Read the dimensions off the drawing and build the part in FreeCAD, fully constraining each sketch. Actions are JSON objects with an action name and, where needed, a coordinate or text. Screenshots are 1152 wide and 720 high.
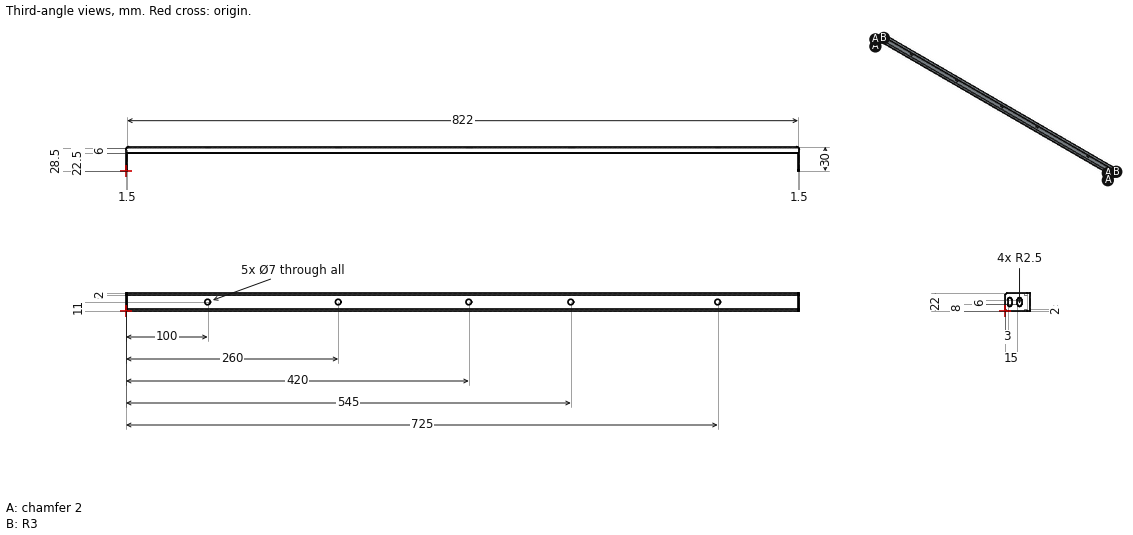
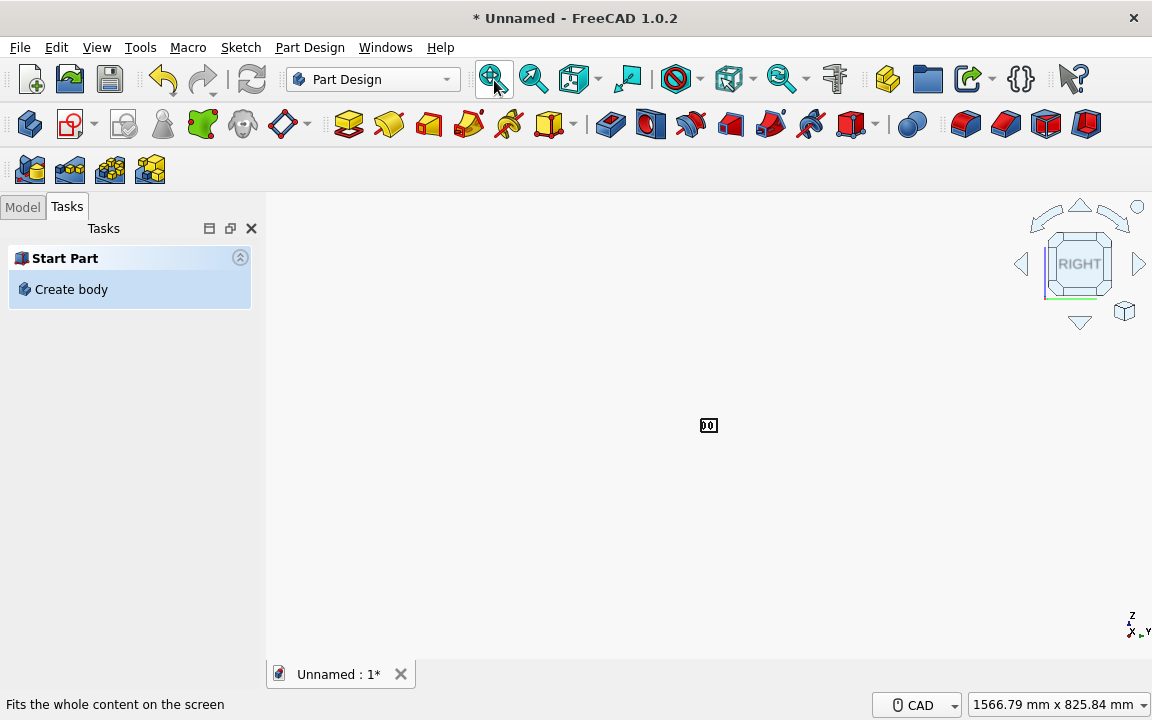
{"action": "left_click", "coordinate": [494, 80]}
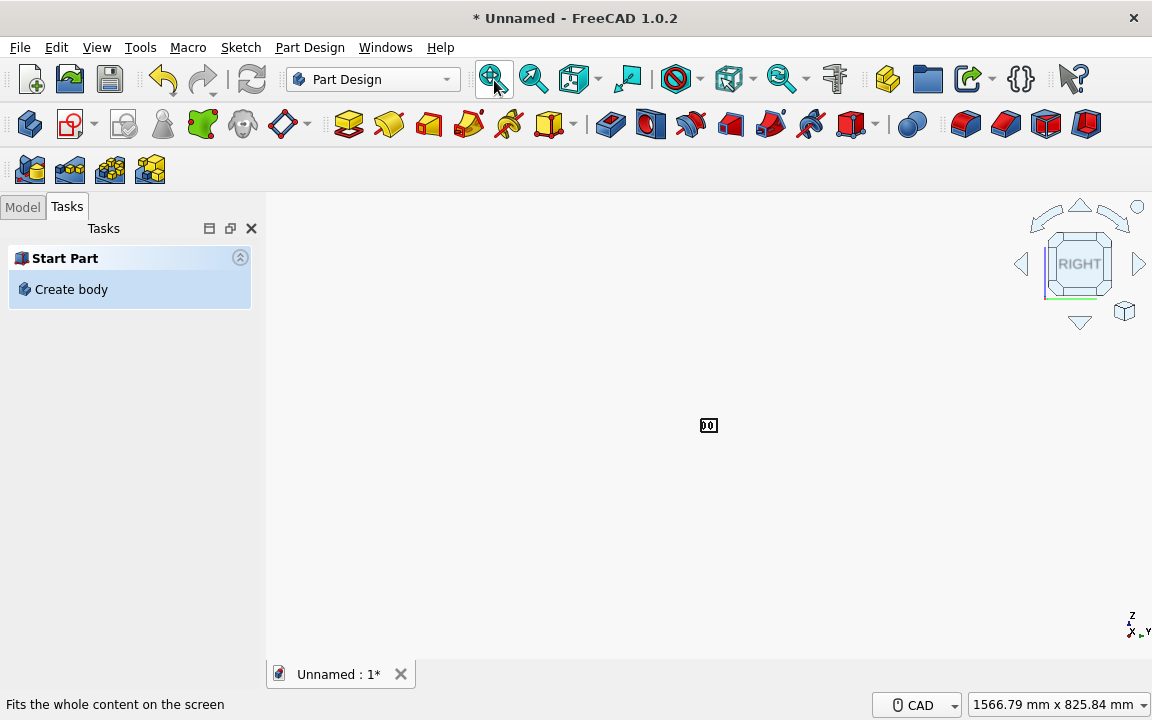
{"action": "scroll", "coordinate": [717, 424], "scroll_direction": "up", "scroll_amount": 6}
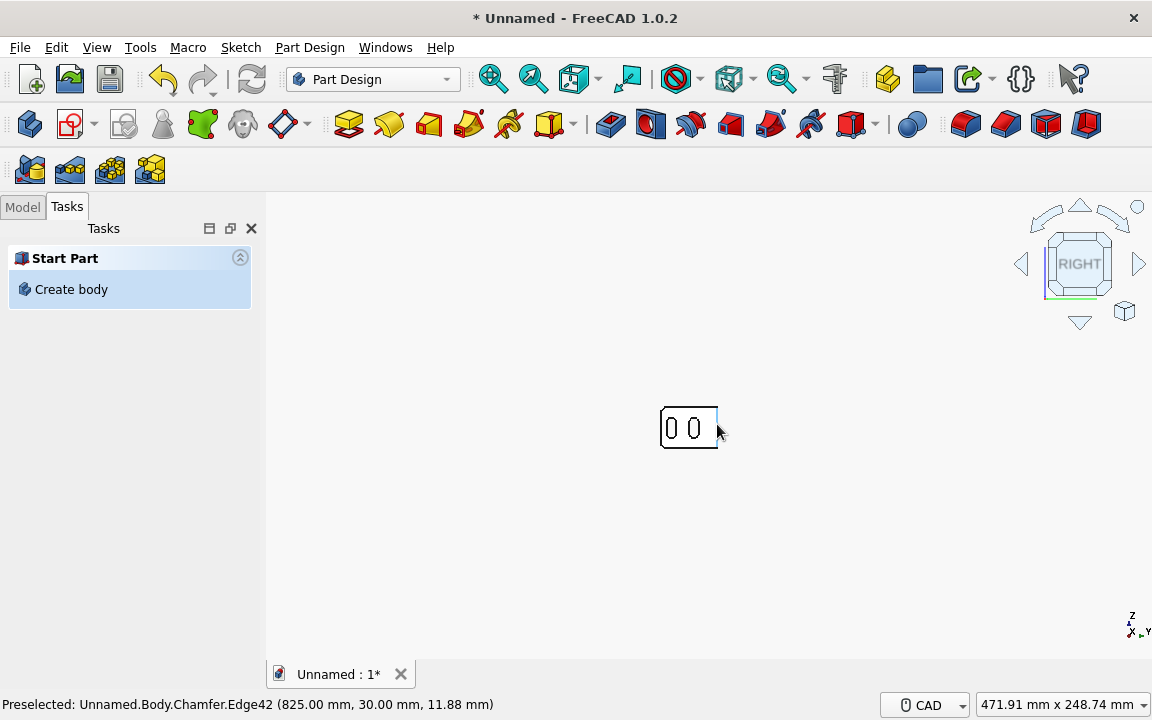
{"action": "left_click", "coordinate": [717, 427]}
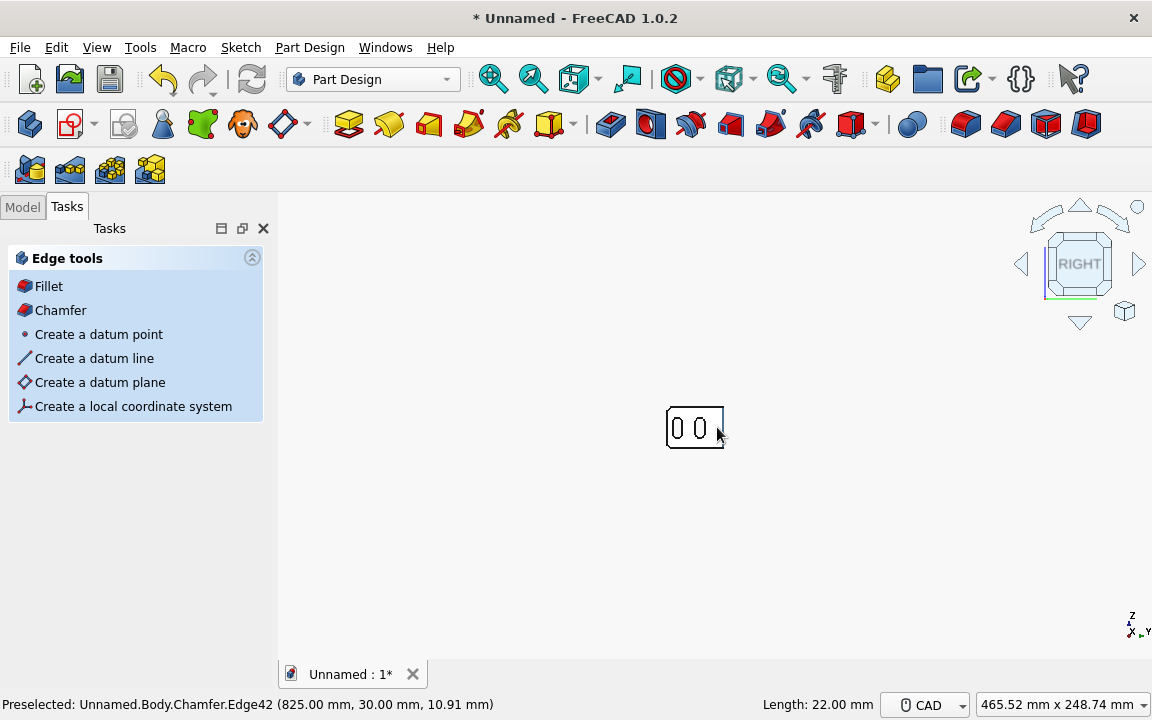
{"action": "left_click", "coordinate": [494, 80]}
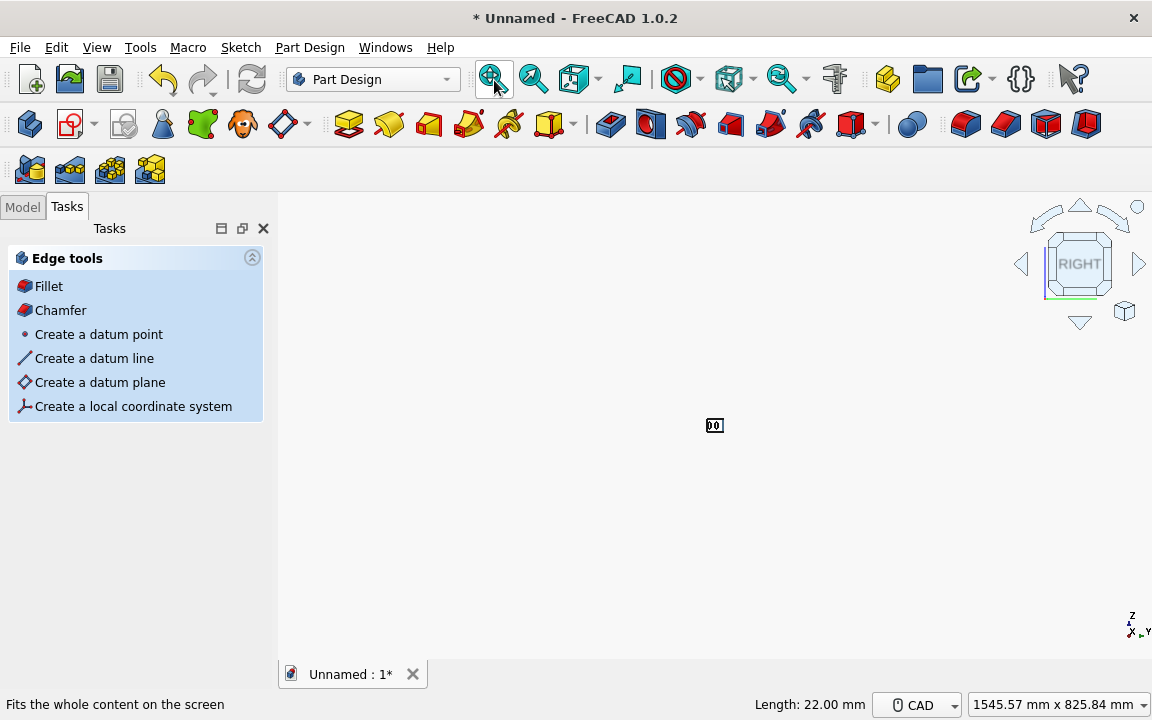
{"action": "key", "text": "5"}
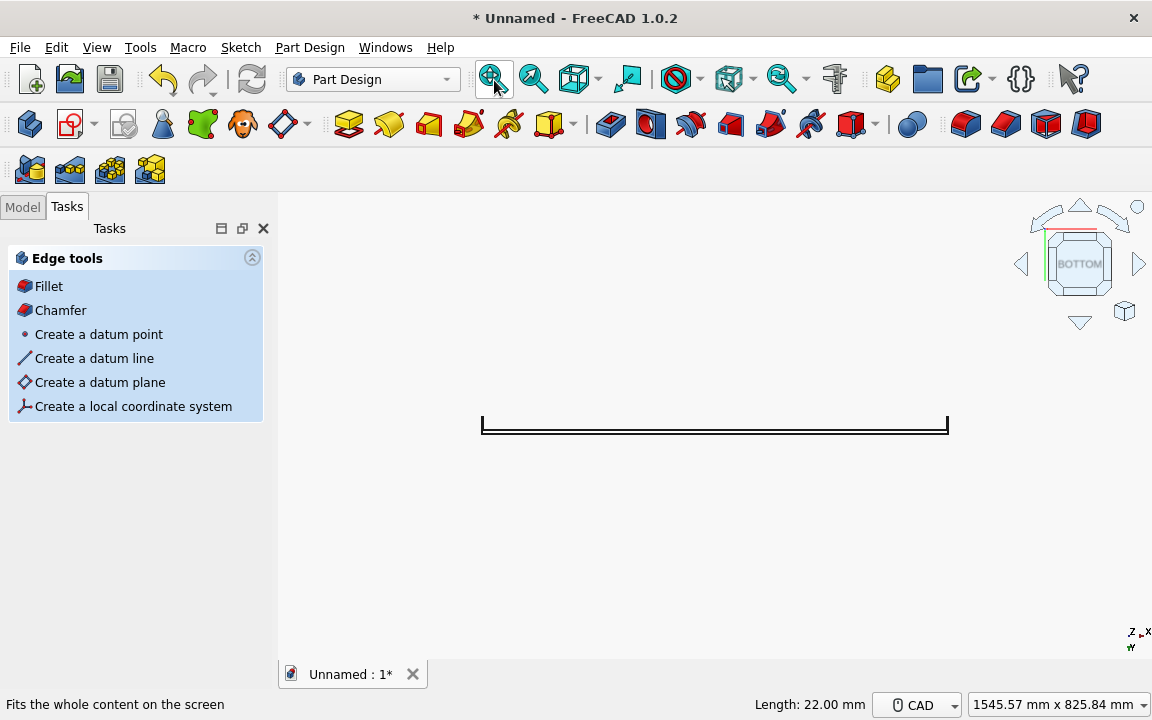
{"action": "scroll", "coordinate": [482, 433], "scroll_direction": "up", "scroll_amount": 6}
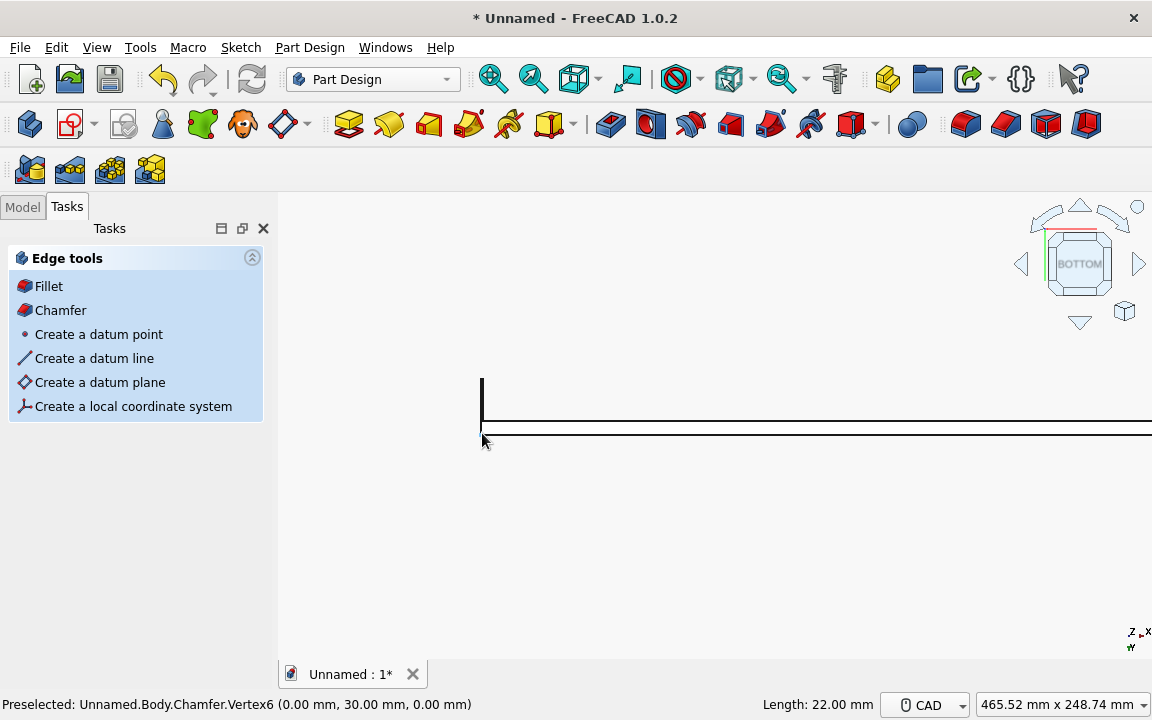
{"action": "left_click", "coordinate": [494, 80]}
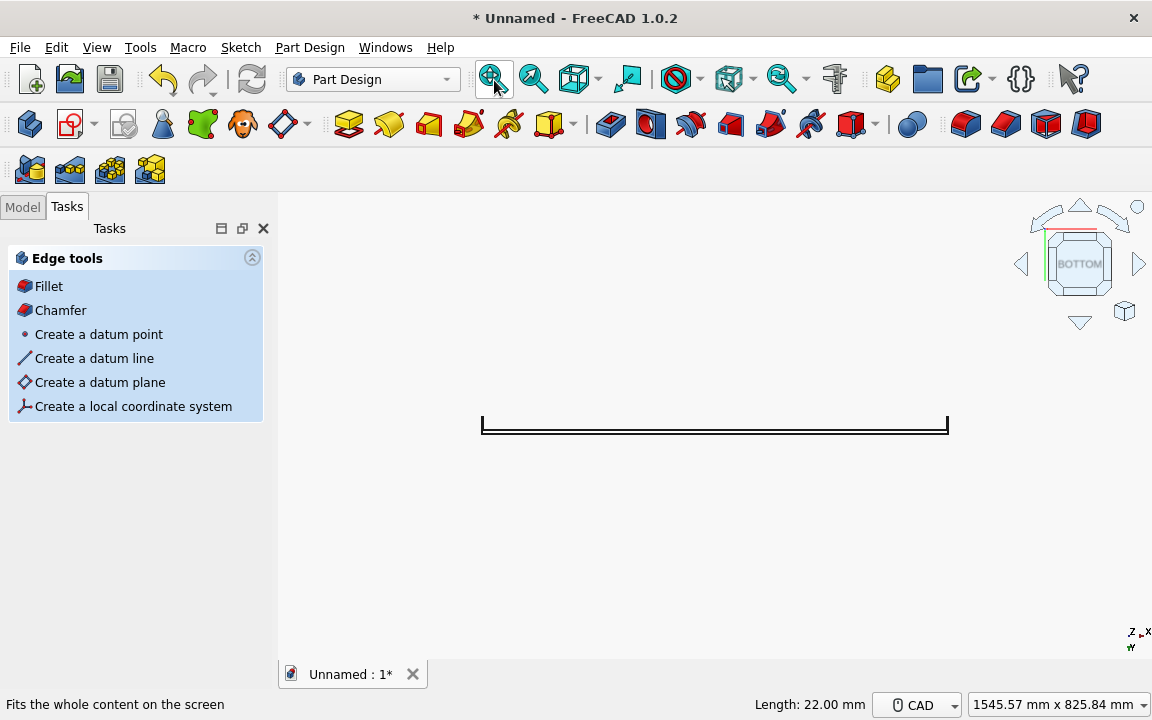
{"action": "key", "text": "4"}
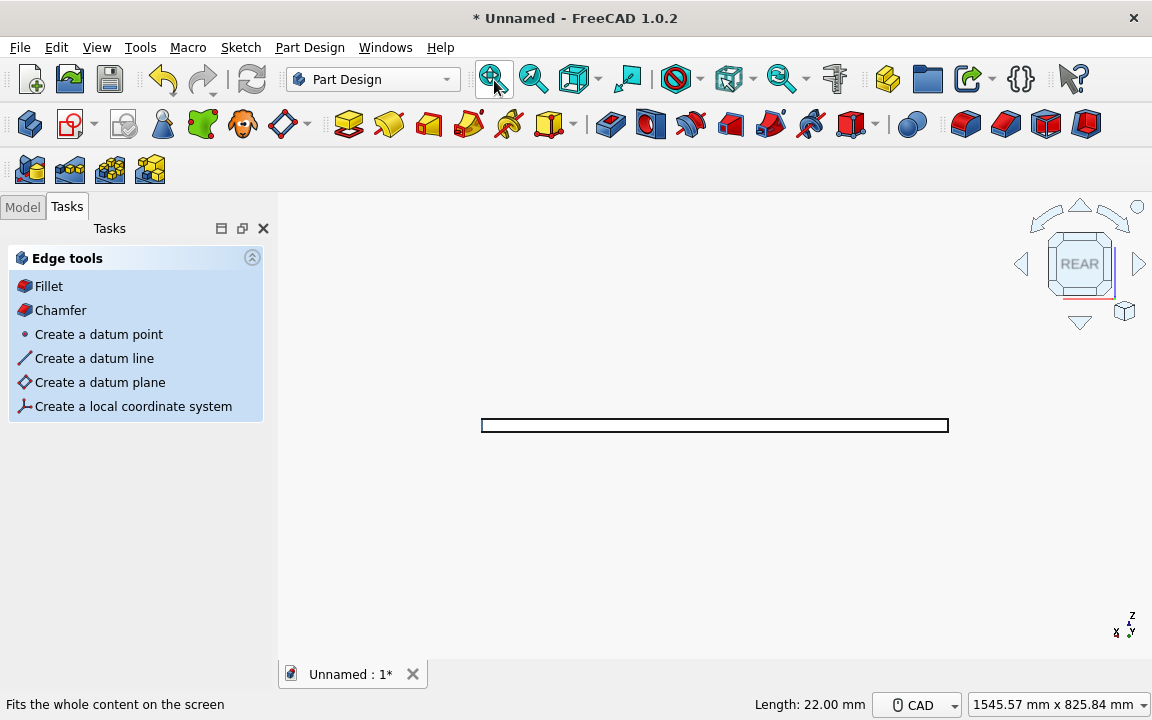
{"action": "scroll", "coordinate": [948, 424], "scroll_direction": "up", "scroll_amount": 6}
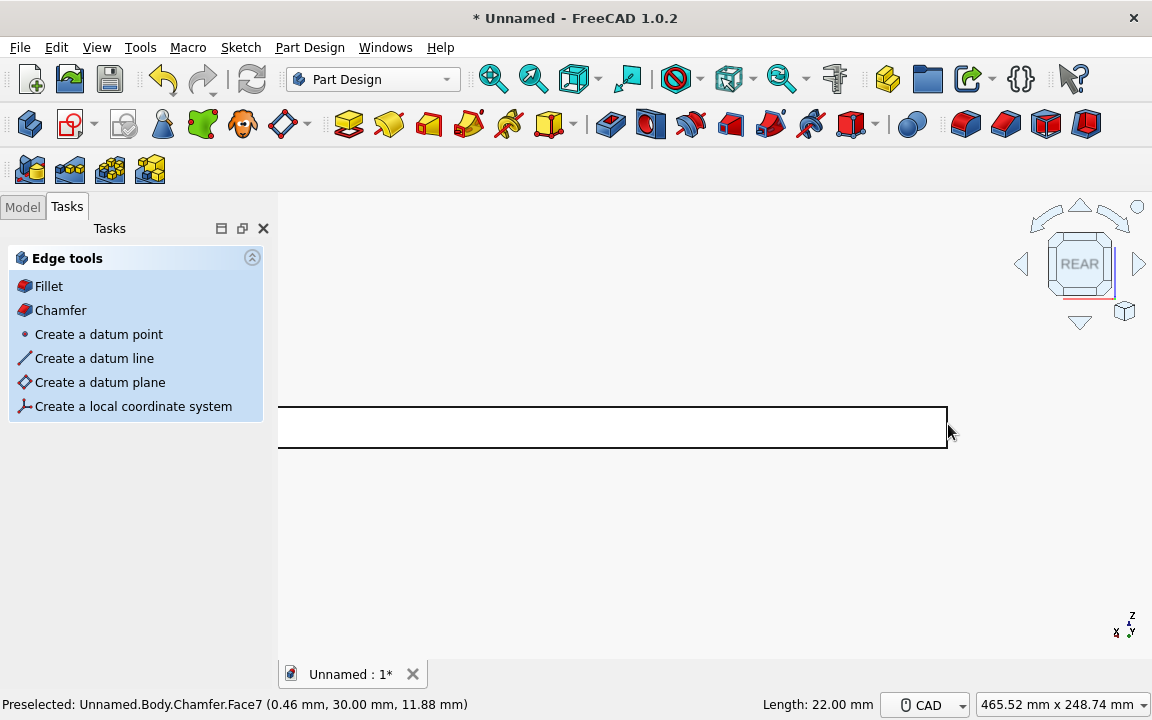
{"action": "left_click", "coordinate": [947, 427], "text": "ctrl"}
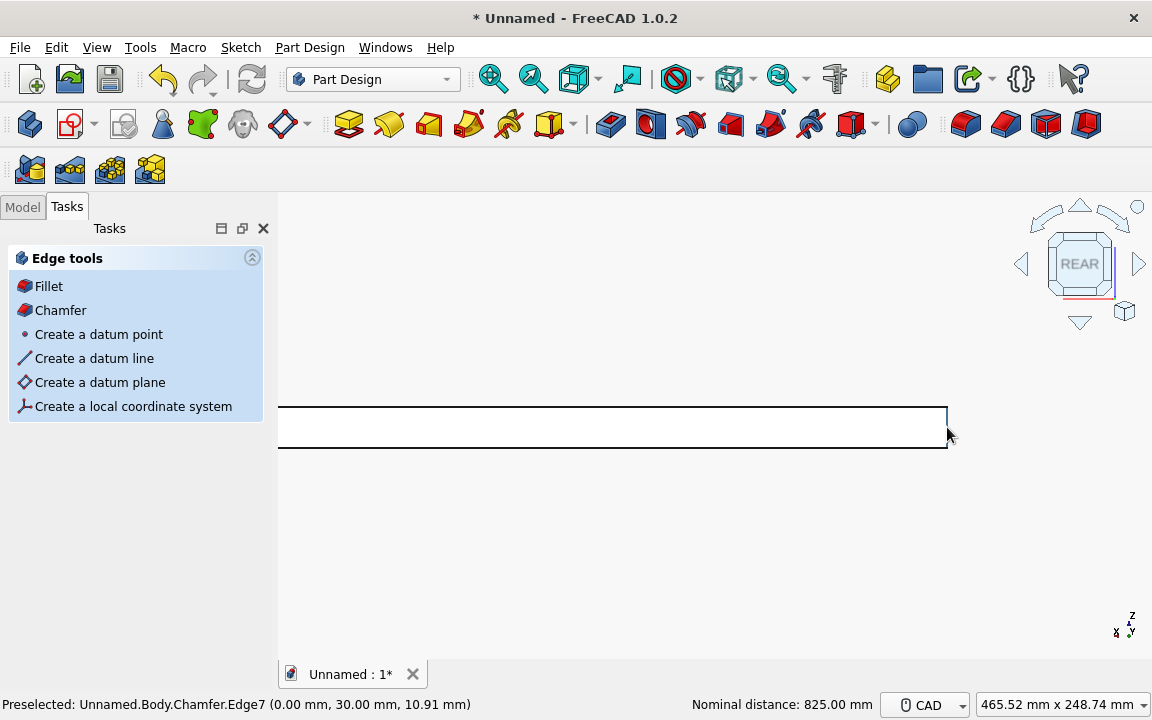
{"action": "left_click", "coordinate": [966, 124]}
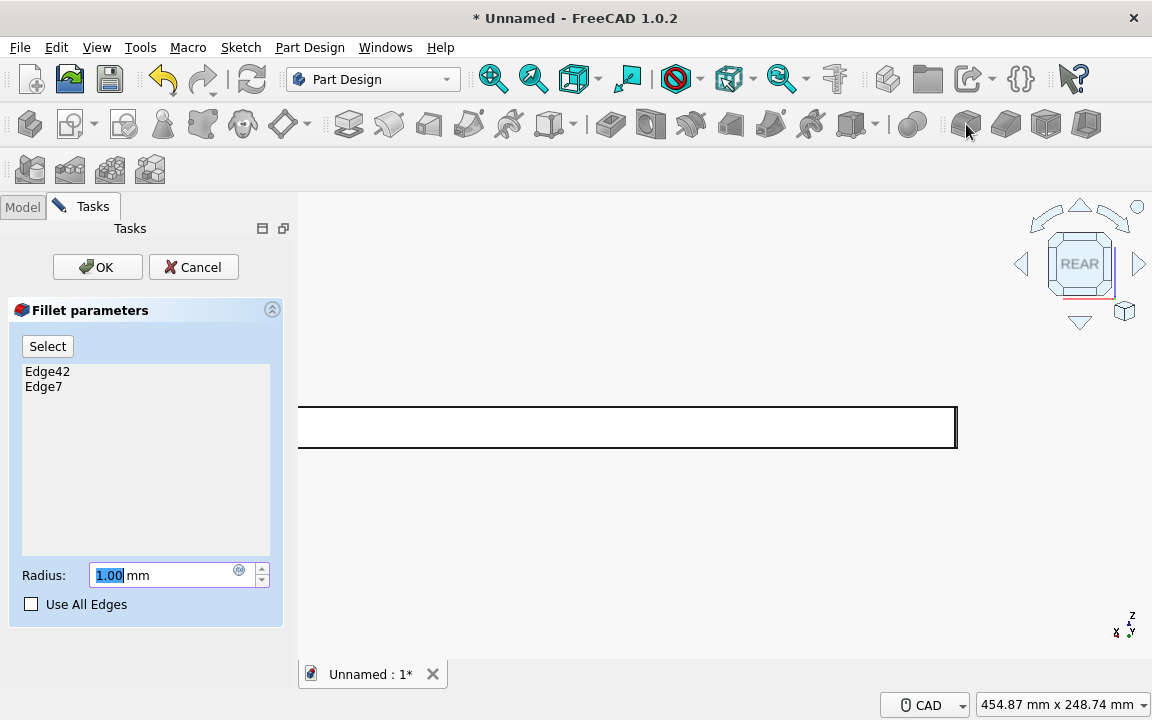
{"action": "type", "text": "3"}
{"action": "key", "text": "Tab"}